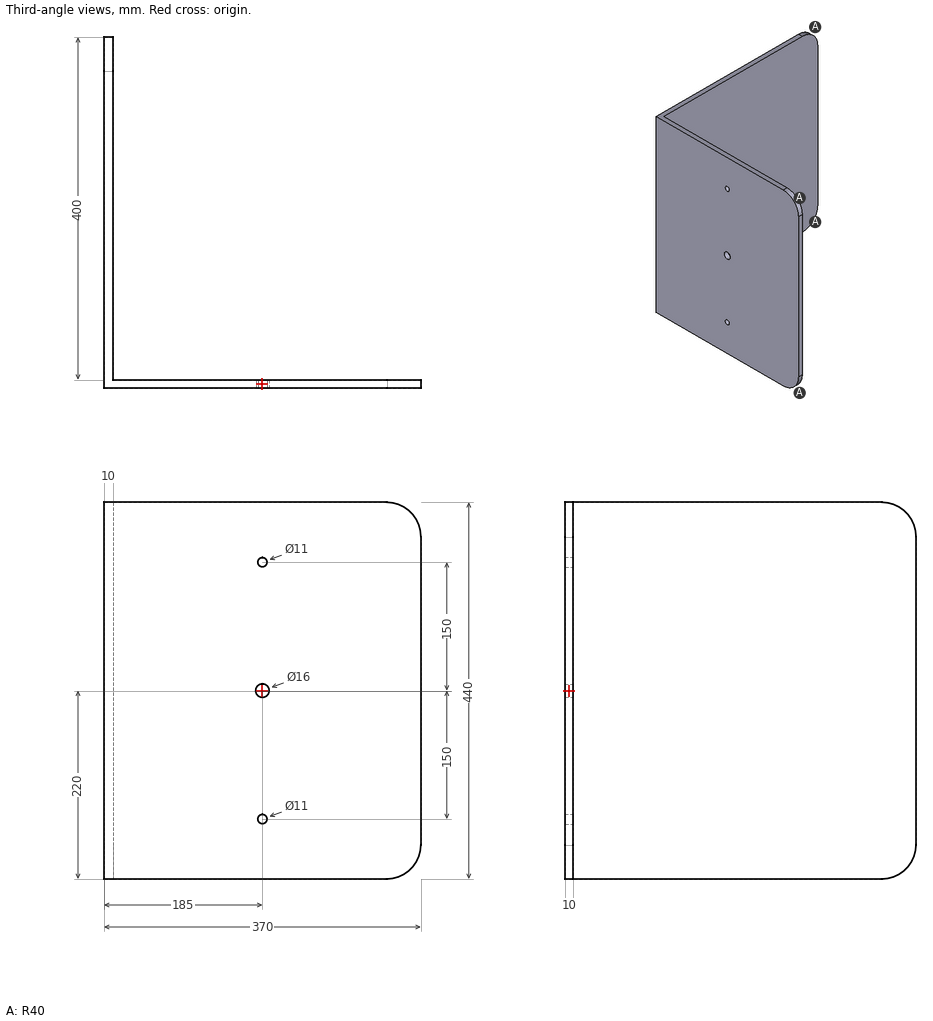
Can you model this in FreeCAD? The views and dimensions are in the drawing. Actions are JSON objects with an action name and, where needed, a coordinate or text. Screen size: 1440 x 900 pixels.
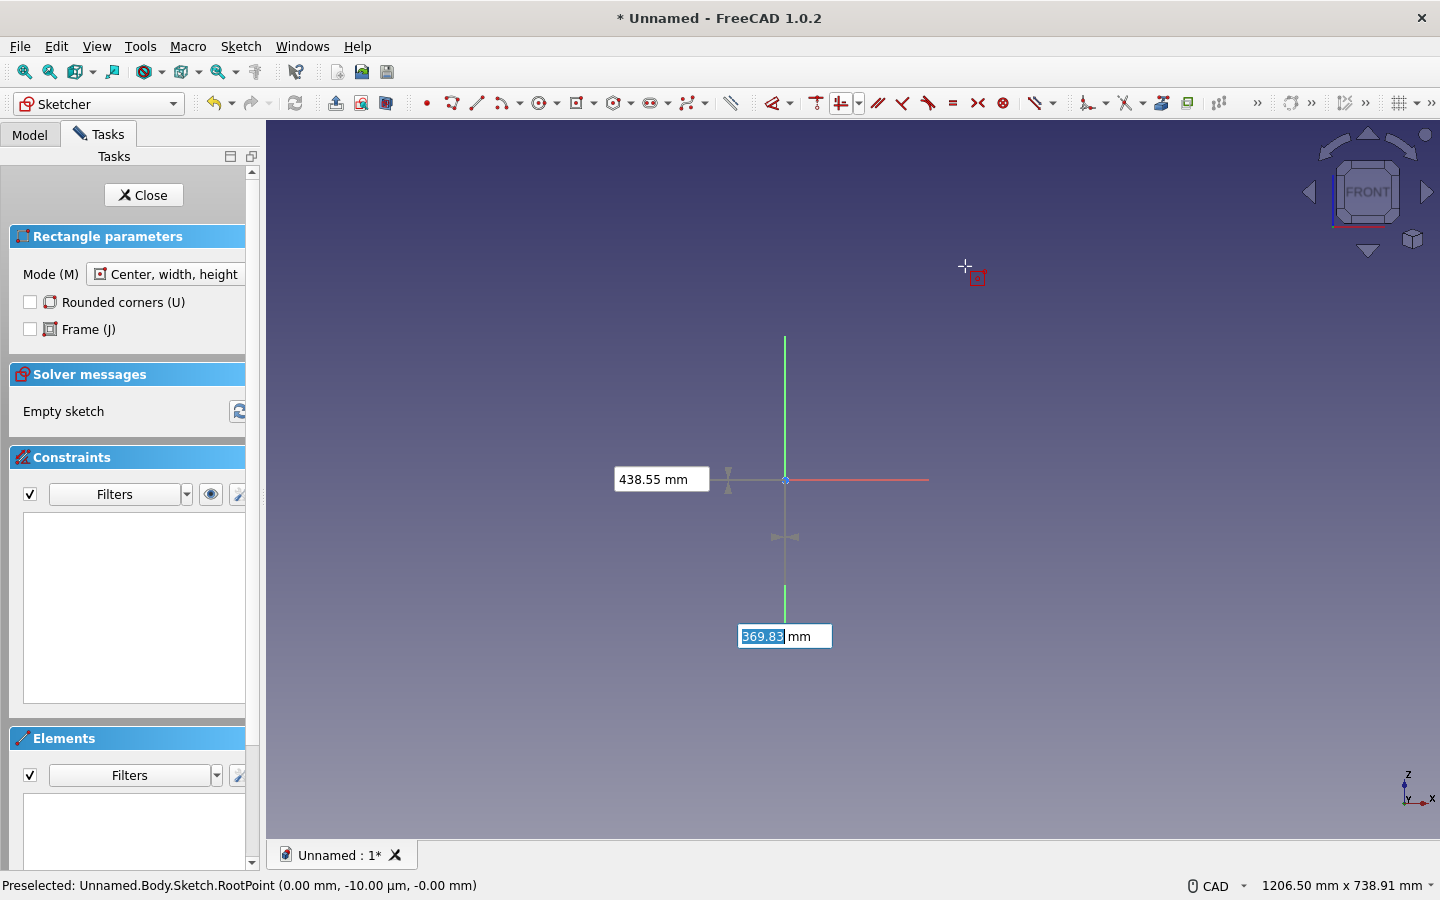
{"action": "type", "text": "370"}
{"action": "key", "text": "Tab"}
{"action": "type", "text": "440"}
{"action": "key", "text": "Return"}
{"action": "key", "text": "Escape"}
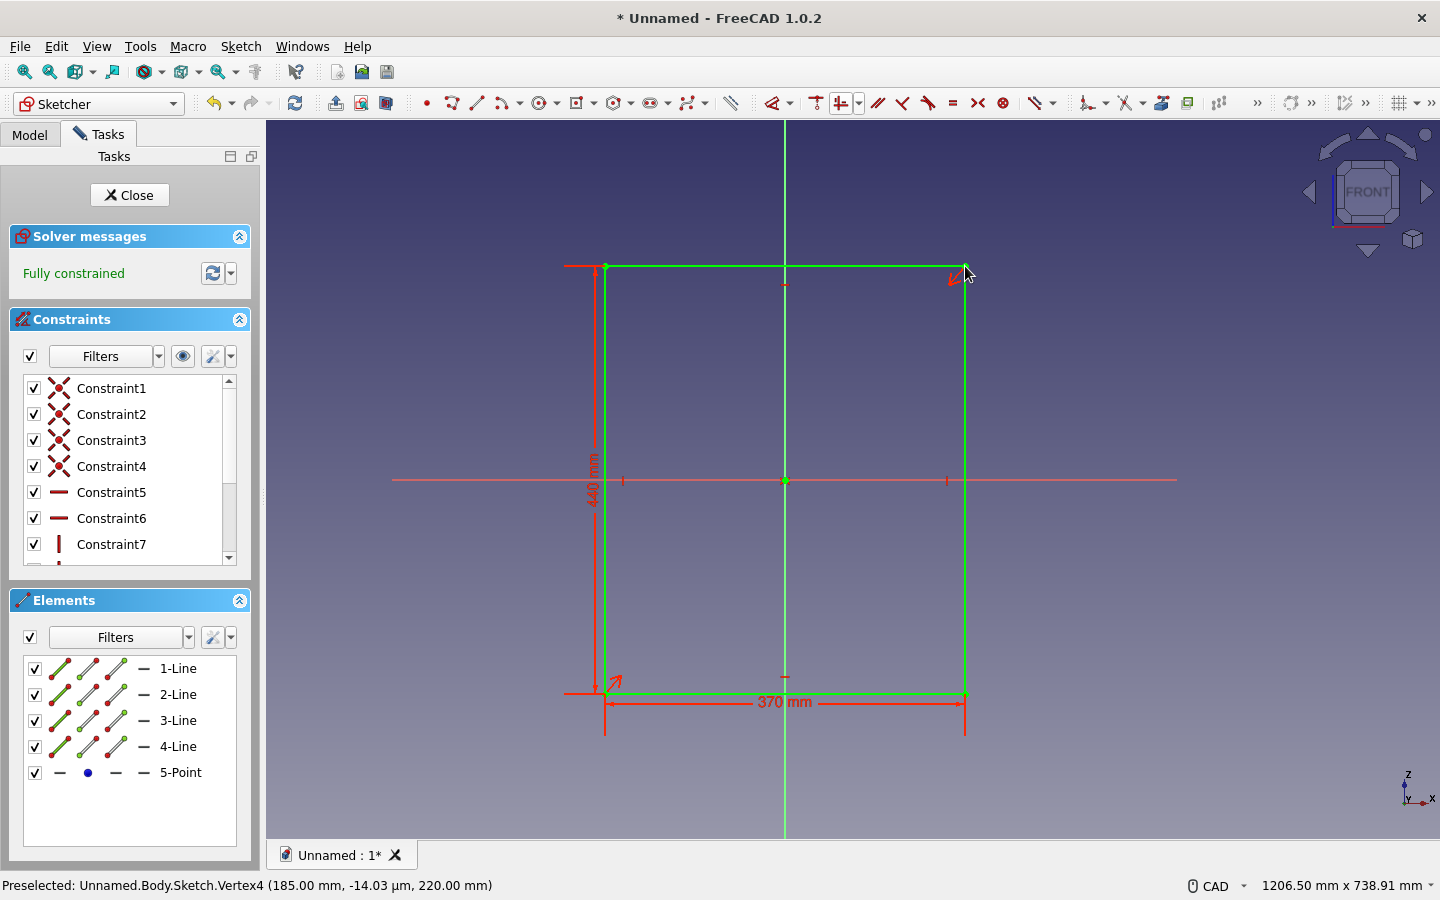
{"action": "left_click", "coordinate": [130, 195]}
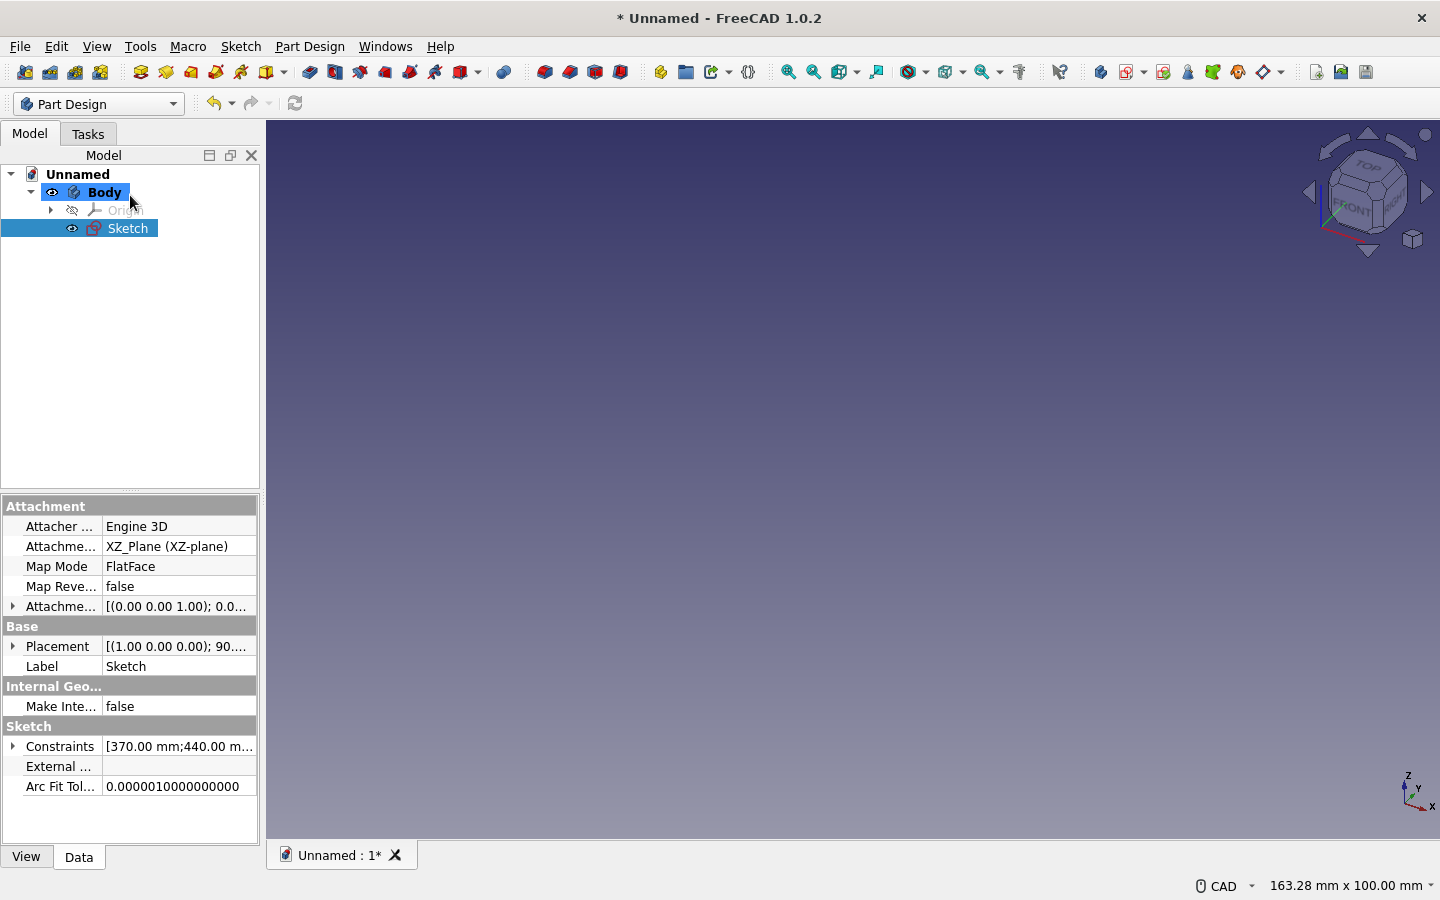
{"action": "left_click", "coordinate": [141, 72]}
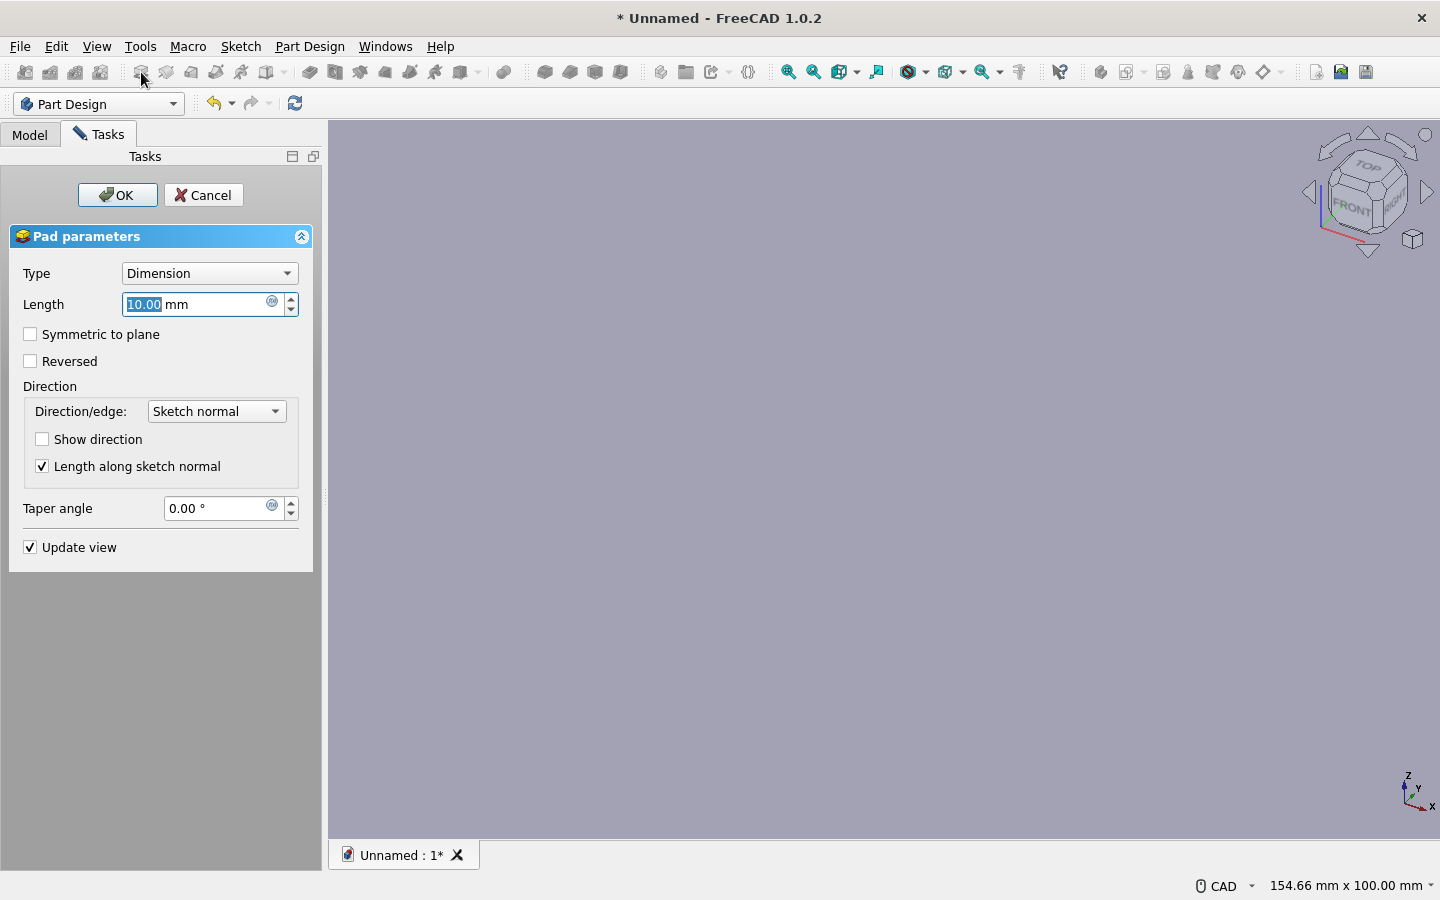
{"action": "type", "text": "10"}
{"action": "key", "text": "Tab"}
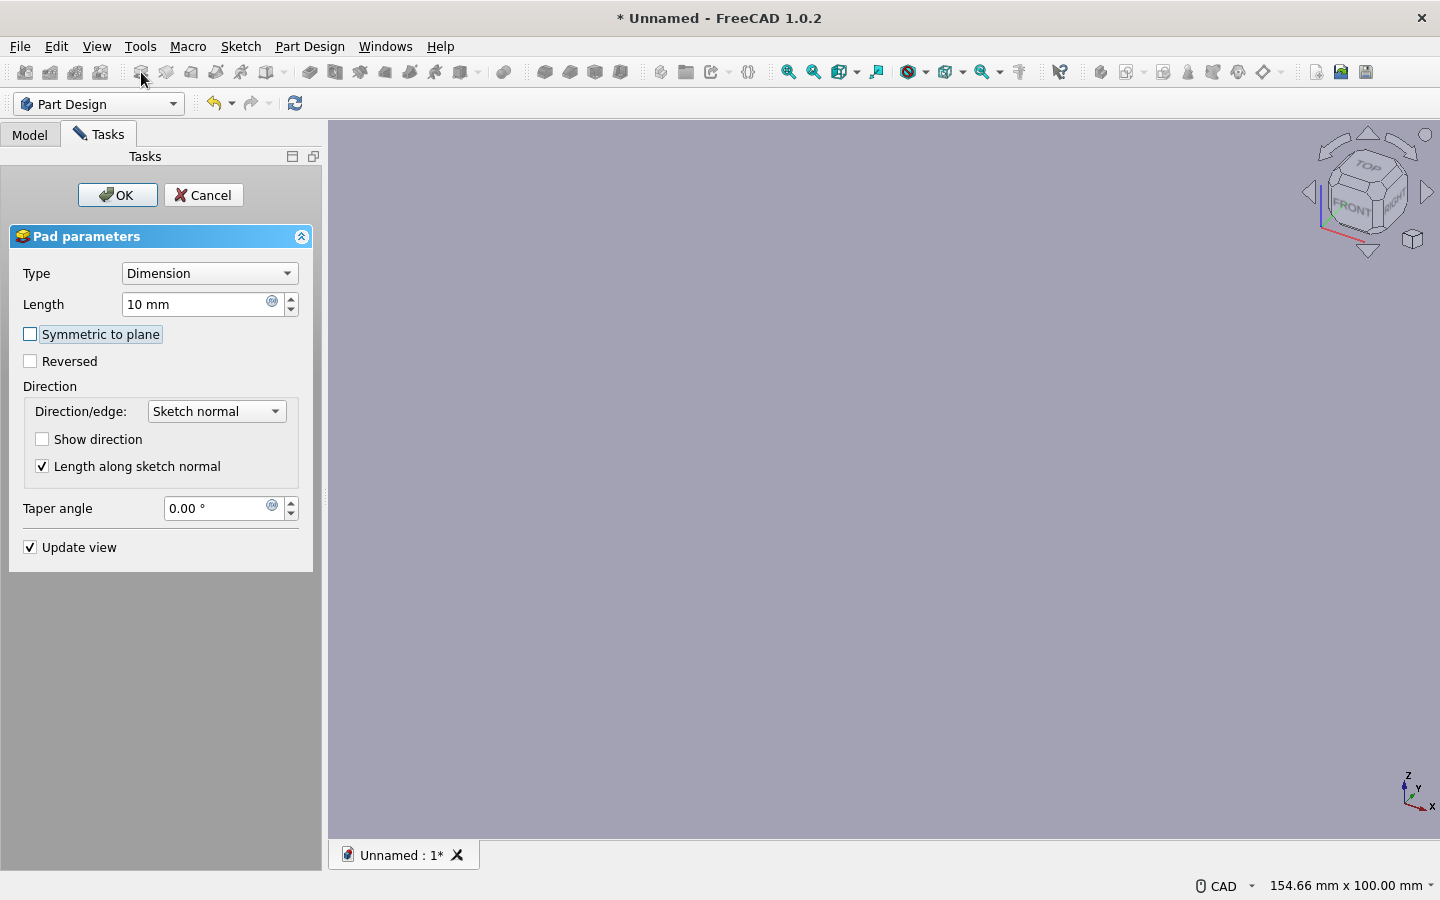
{"action": "left_click", "coordinate": [31, 334]}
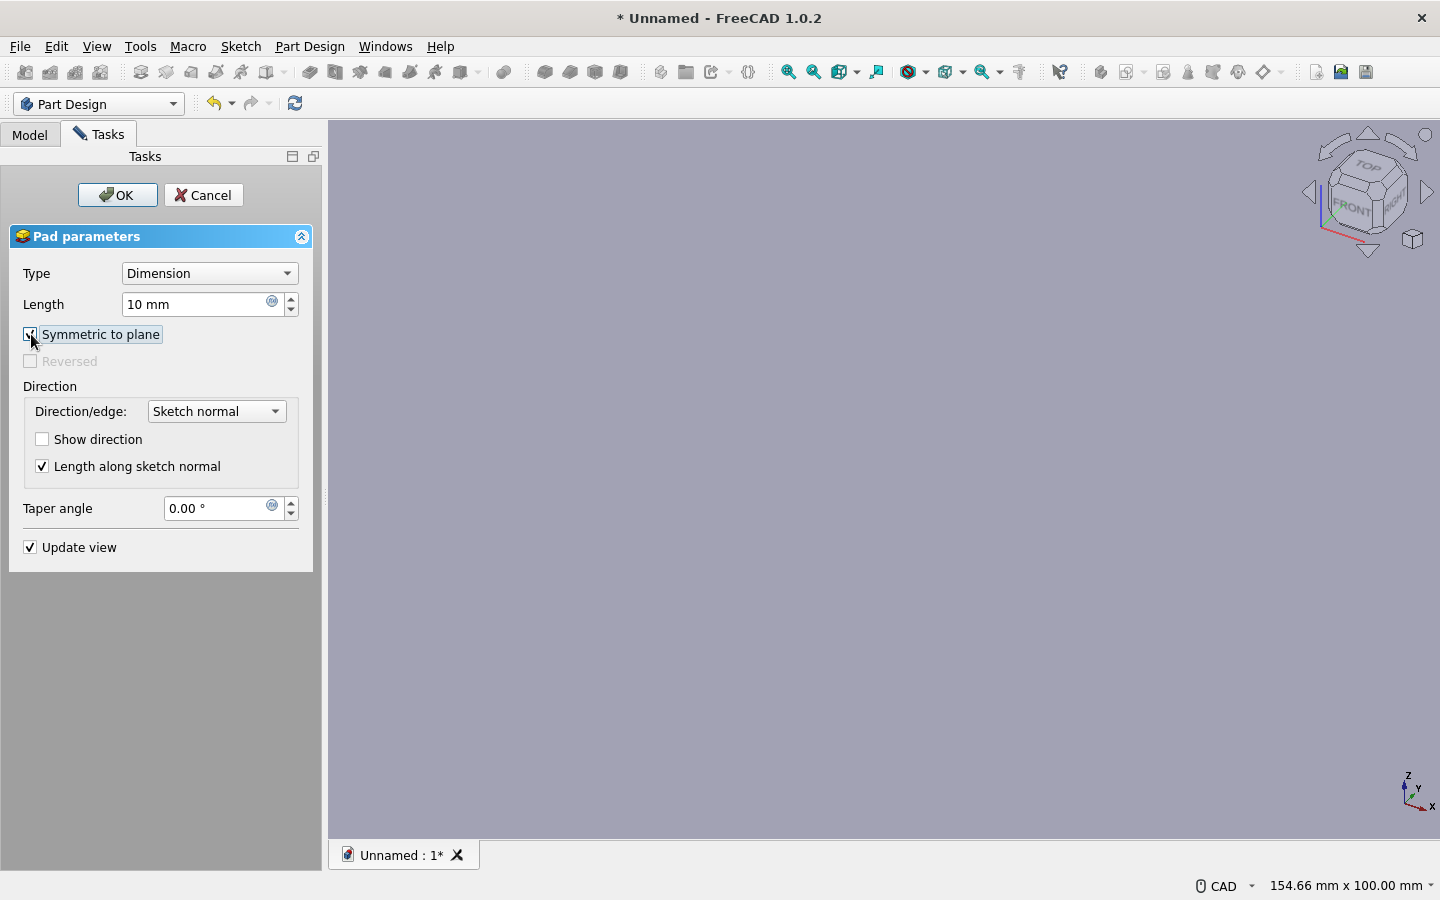
{"action": "left_click", "coordinate": [118, 195]}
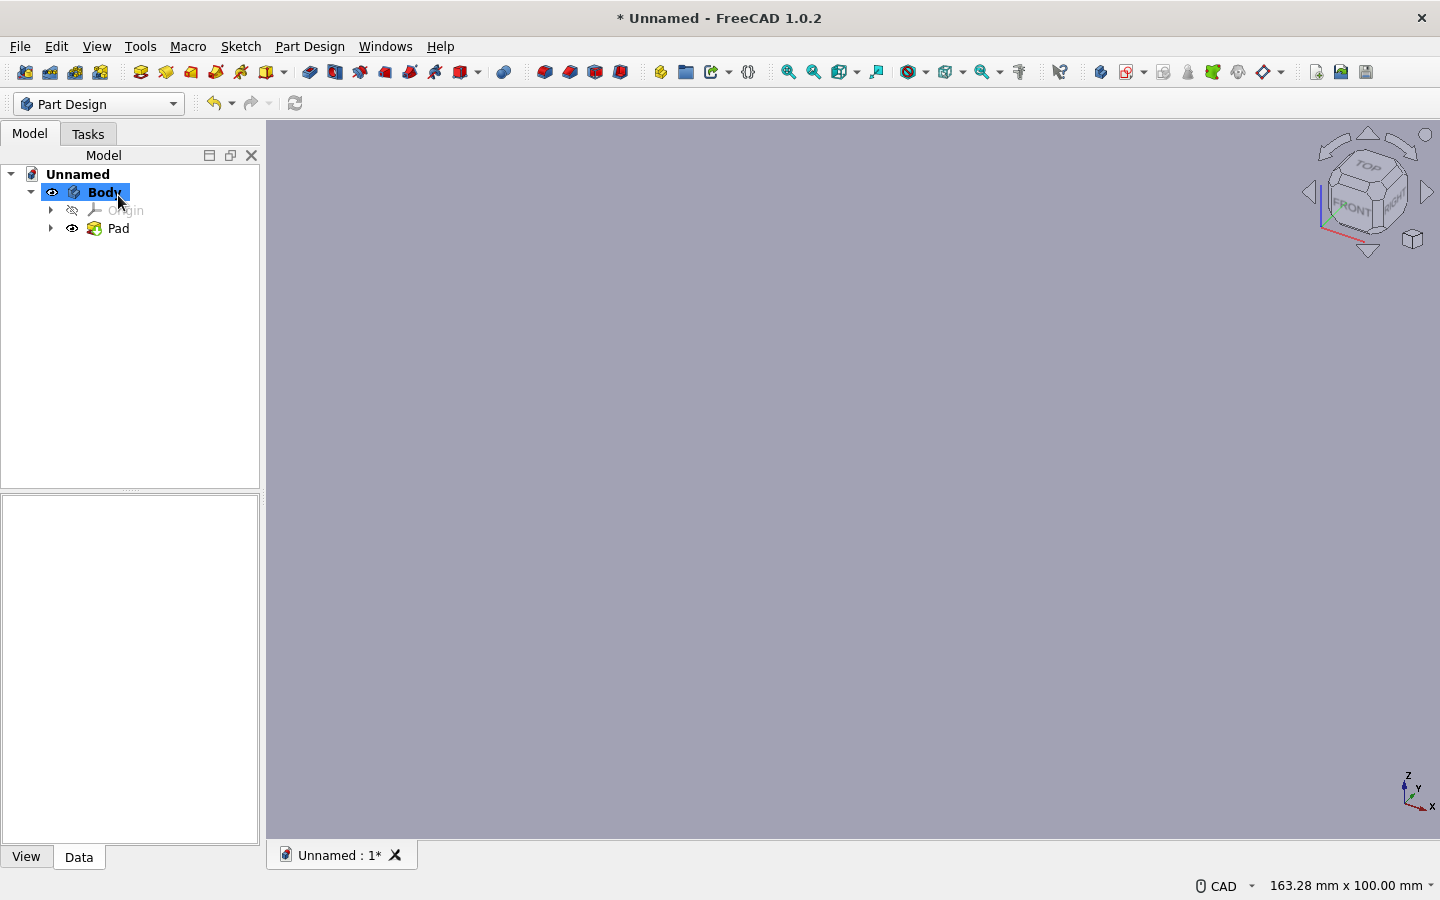
{"action": "left_click", "coordinate": [789, 72]}